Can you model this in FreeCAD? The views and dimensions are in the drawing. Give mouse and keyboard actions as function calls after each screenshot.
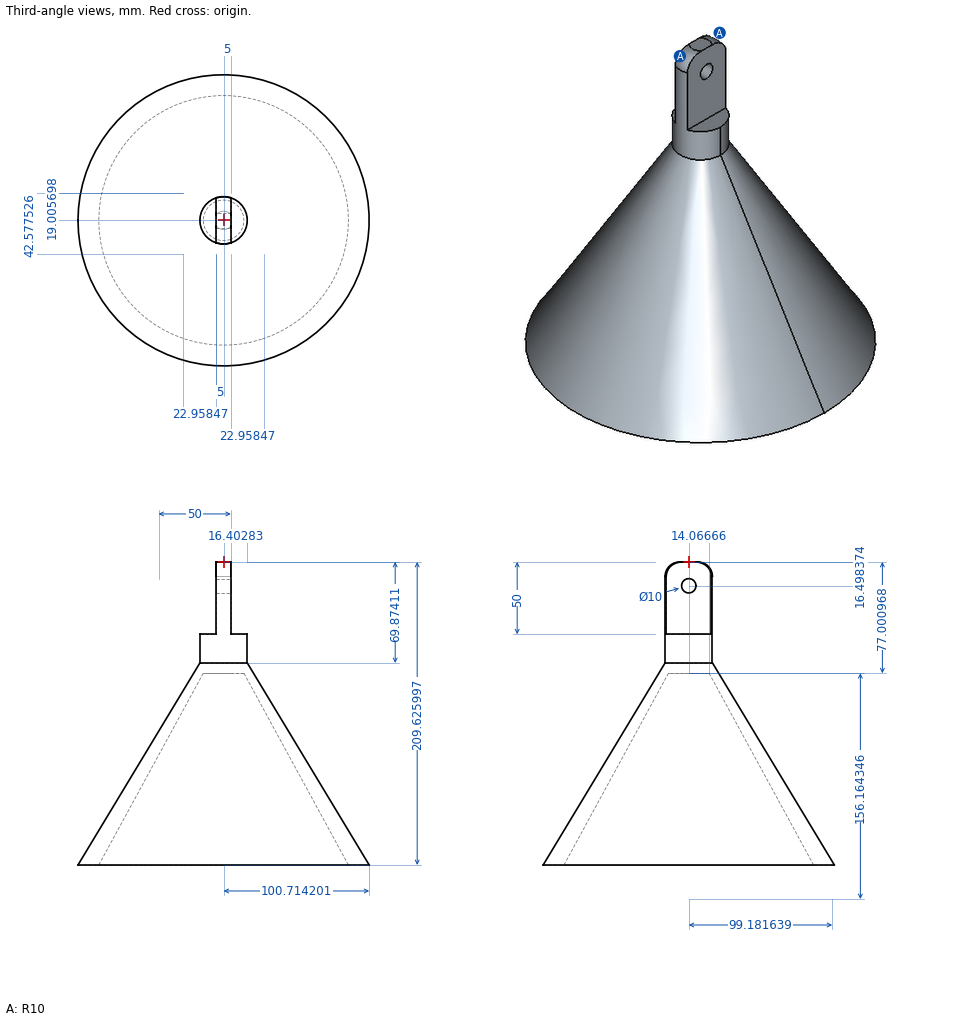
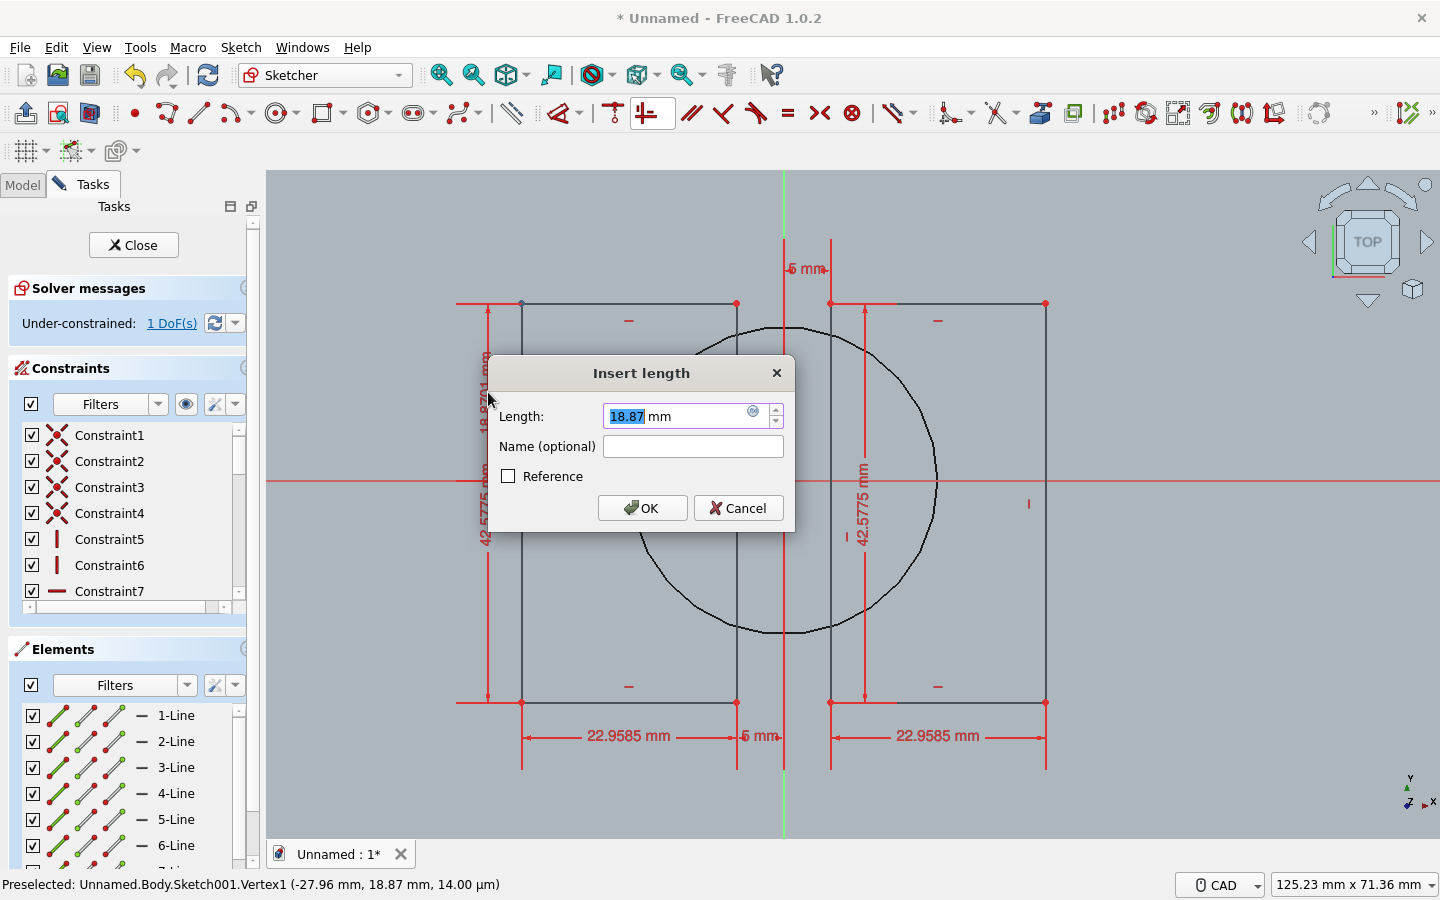
text(19.005698)
key(Return)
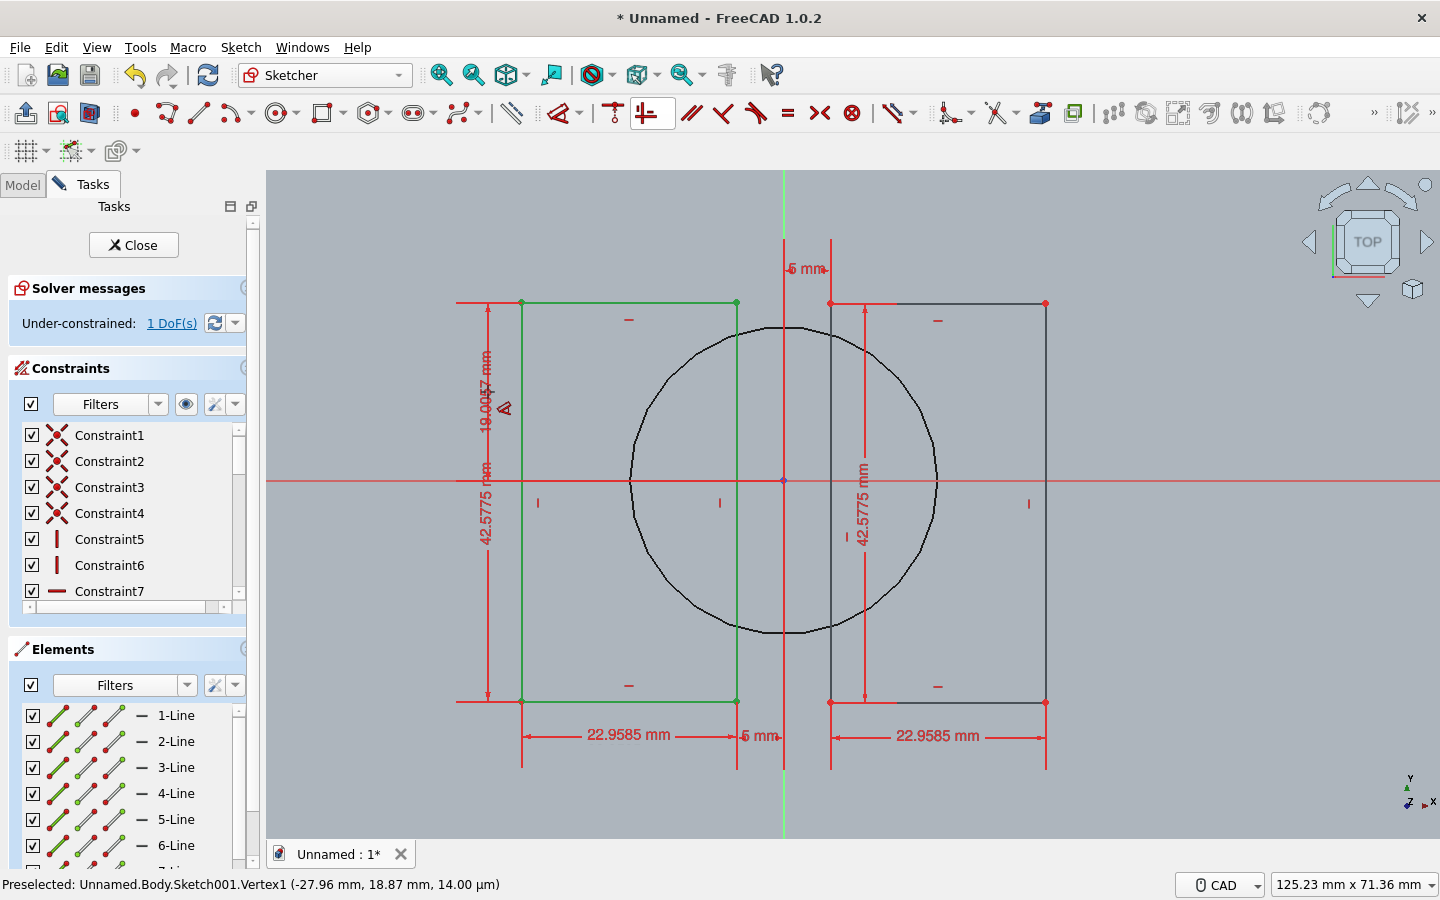
click(831, 304)
click(865, 392)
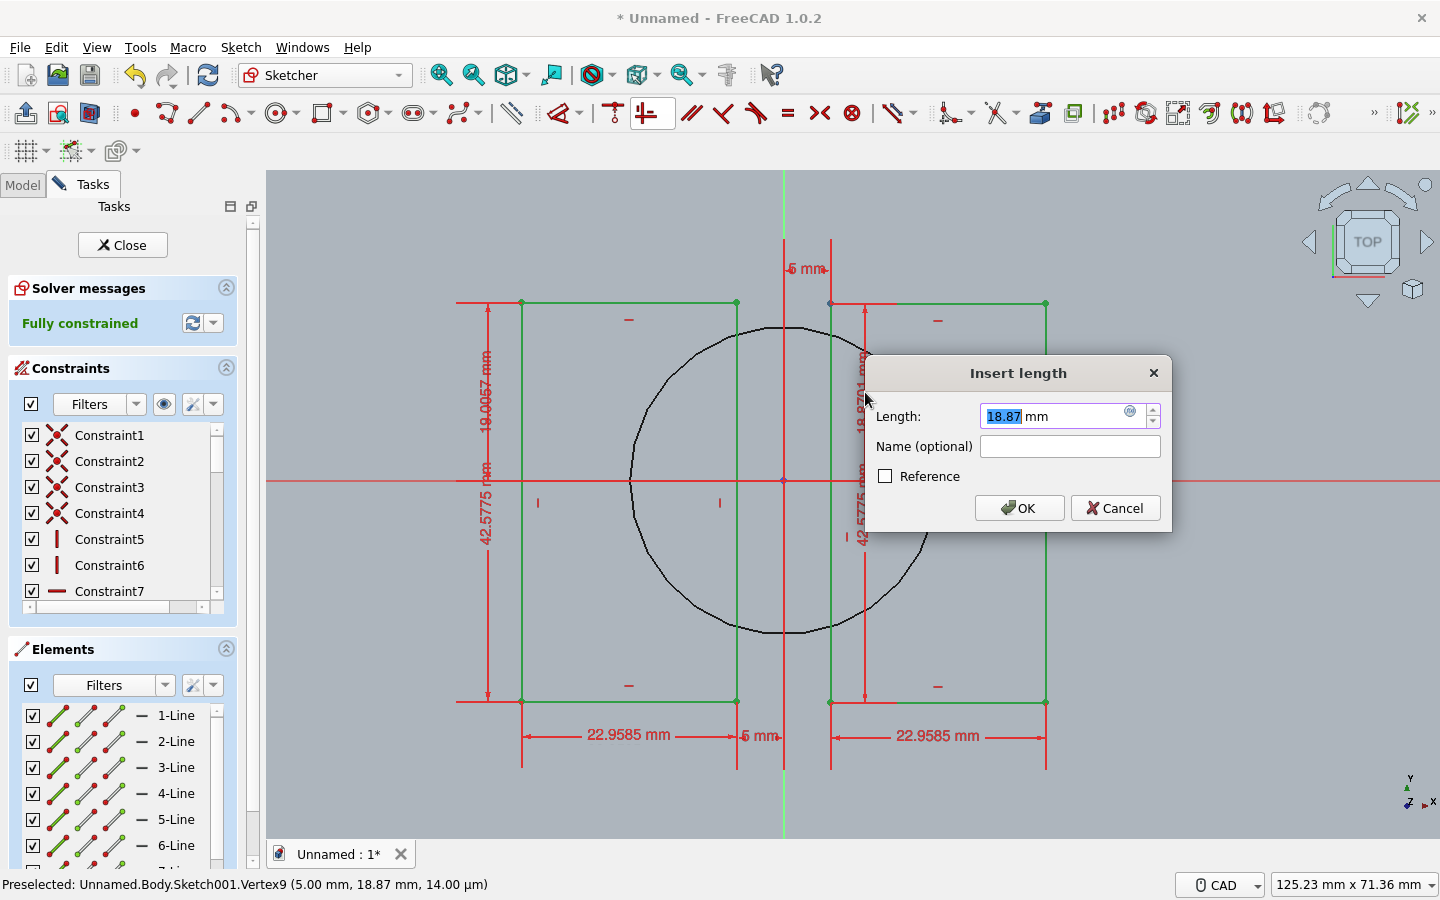
text(19.005698)
key(Return)
key(Escape)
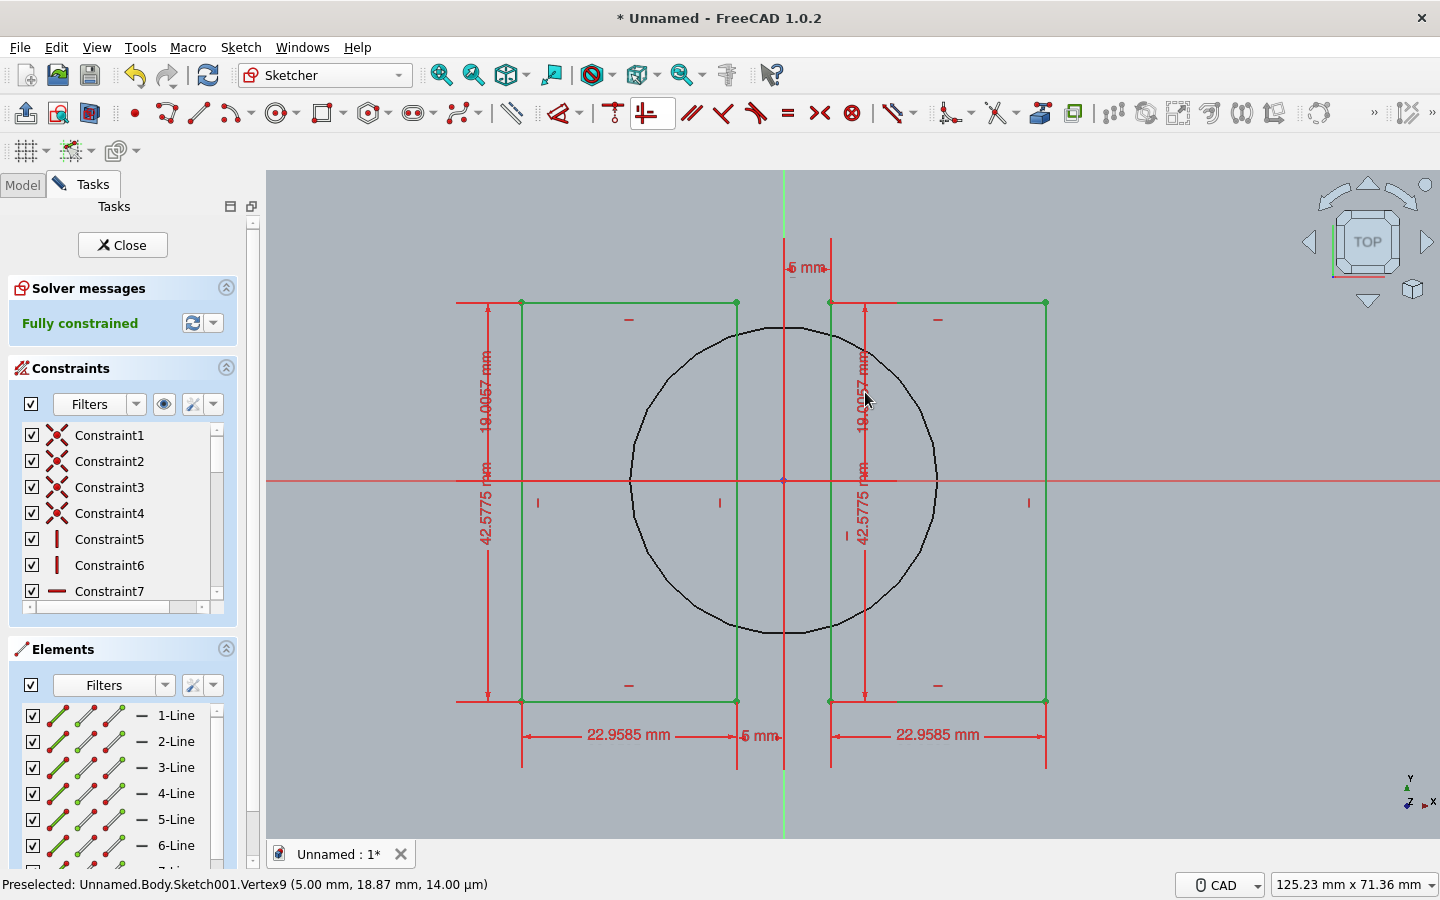
click(123, 245)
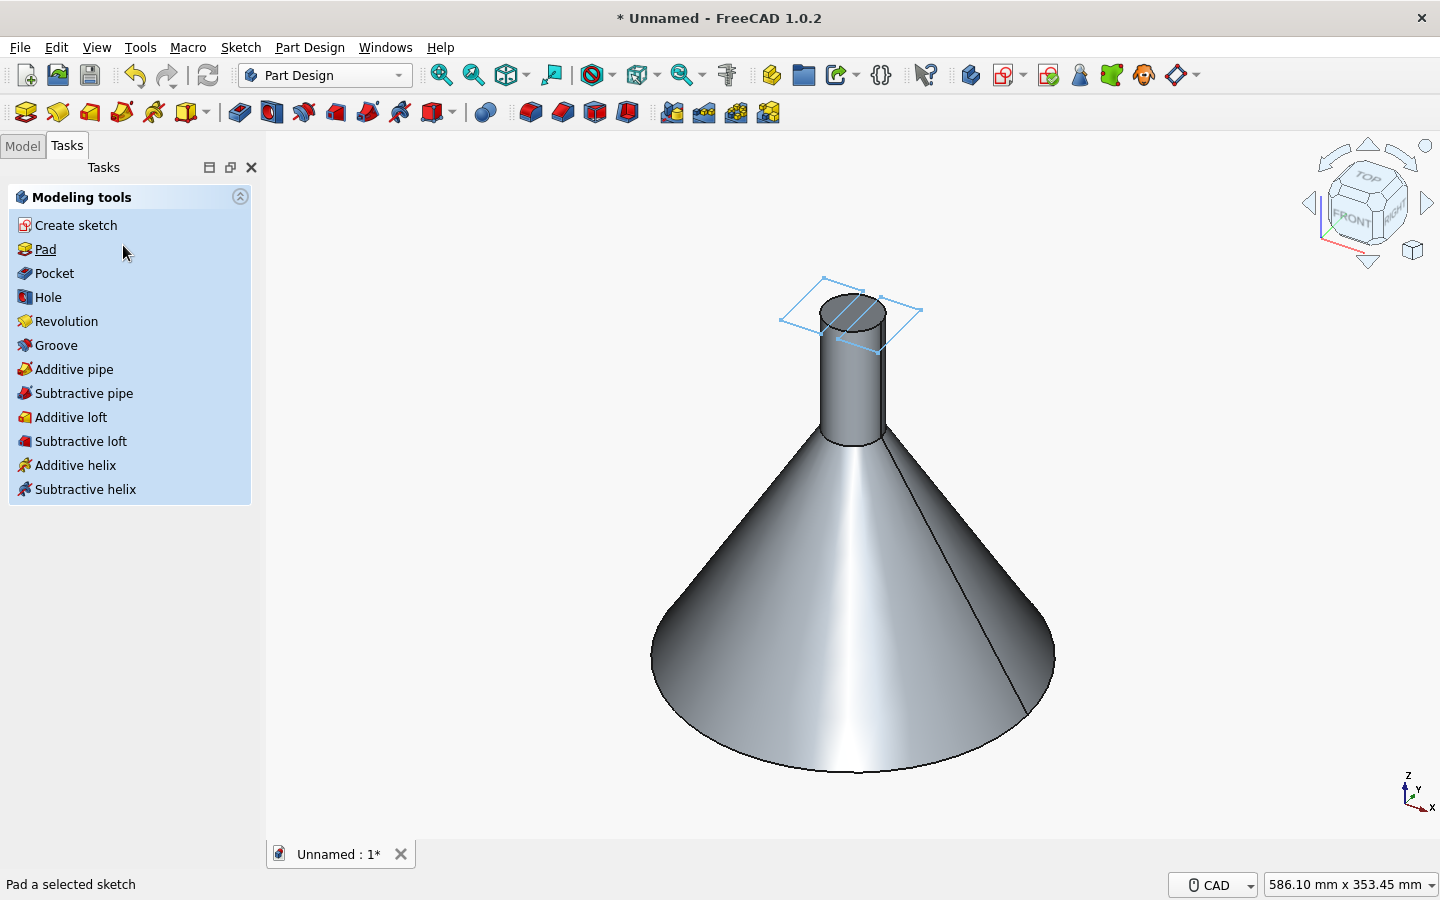
click(240, 112)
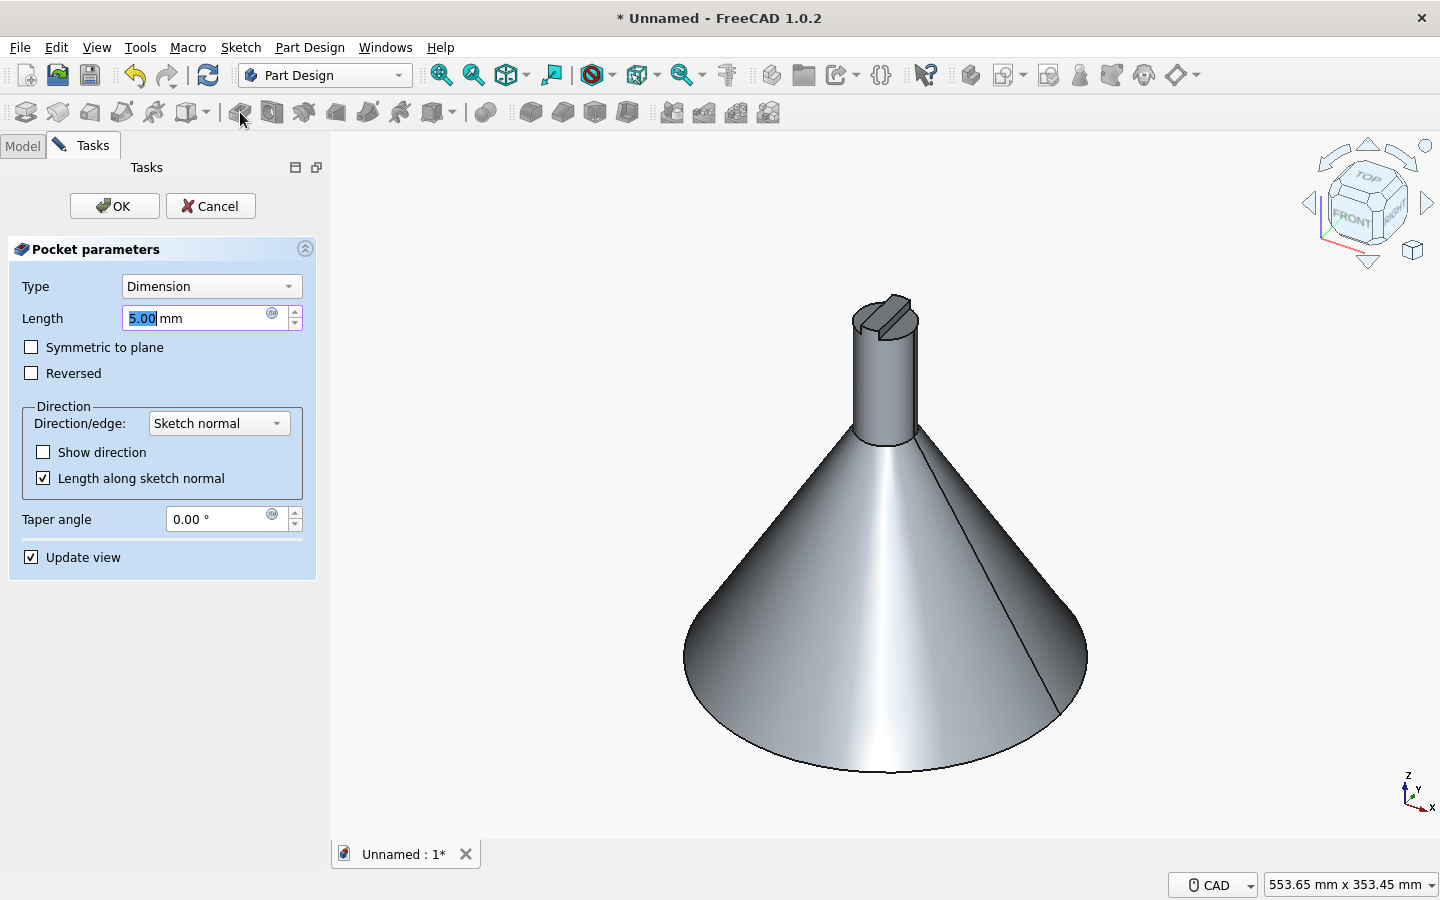
text(50)
key(Tab)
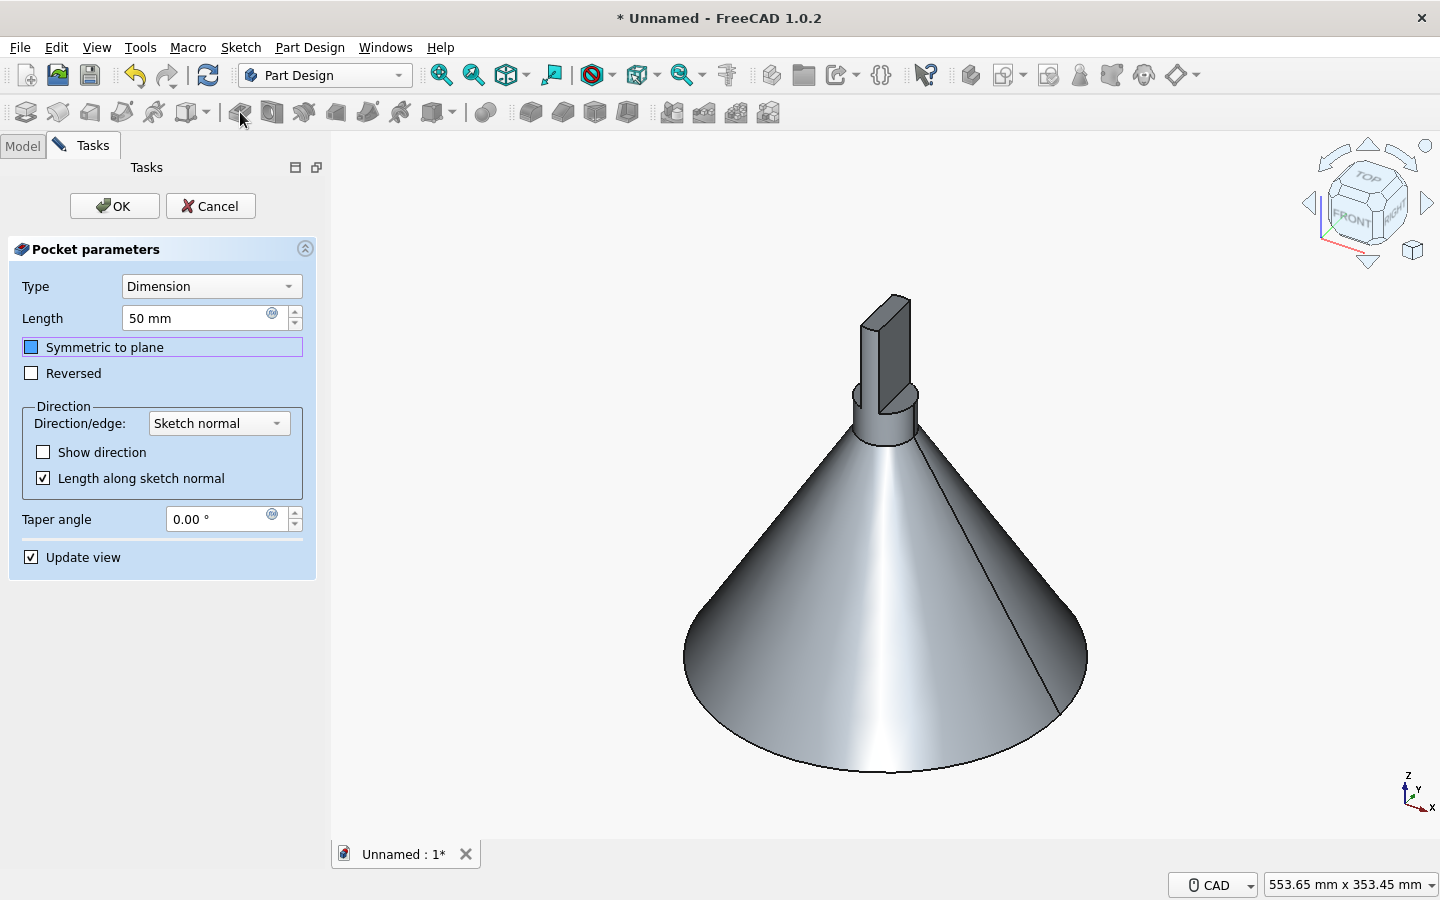
click(115, 206)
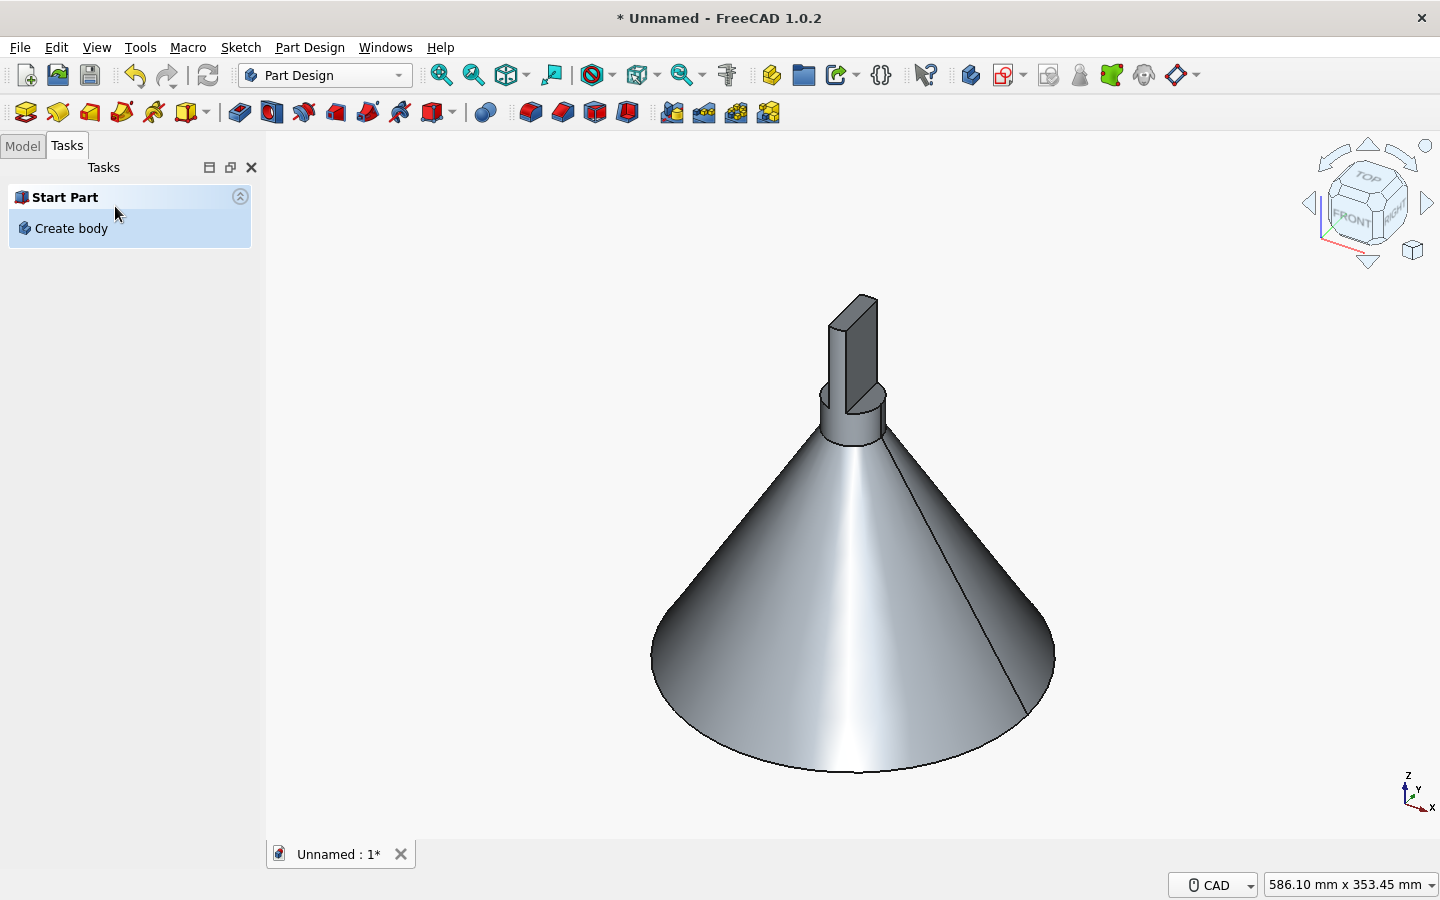
click(862, 344)